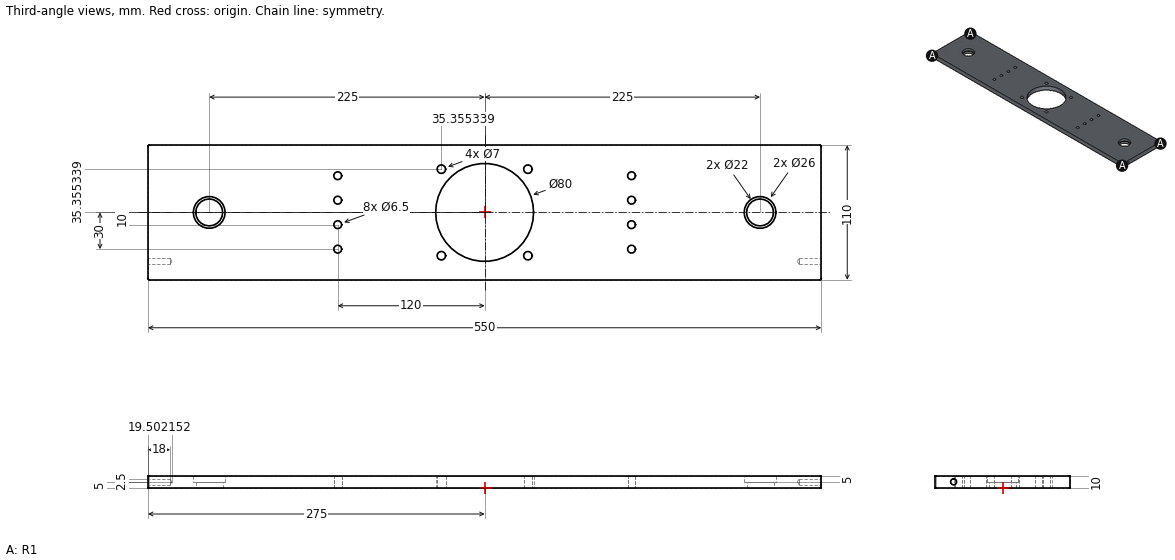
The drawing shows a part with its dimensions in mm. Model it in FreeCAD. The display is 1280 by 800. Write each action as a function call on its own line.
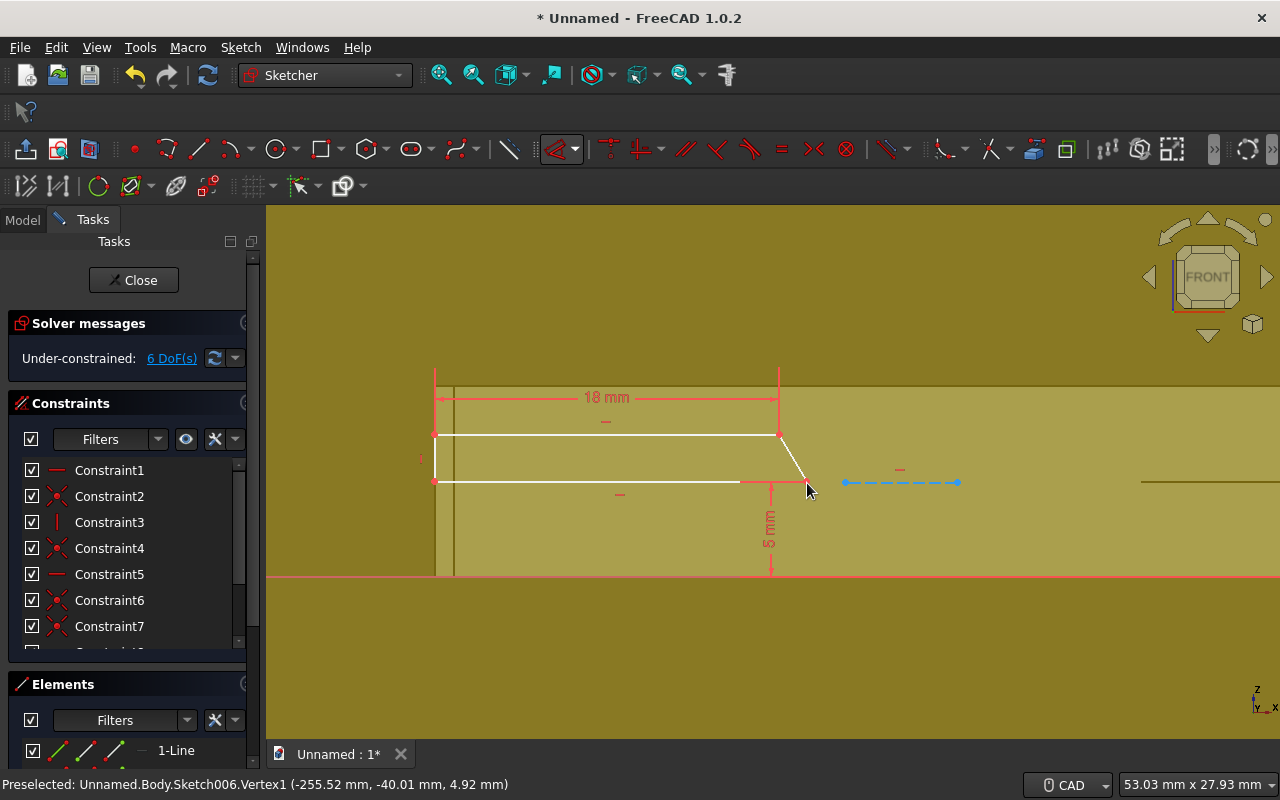
click(845, 483)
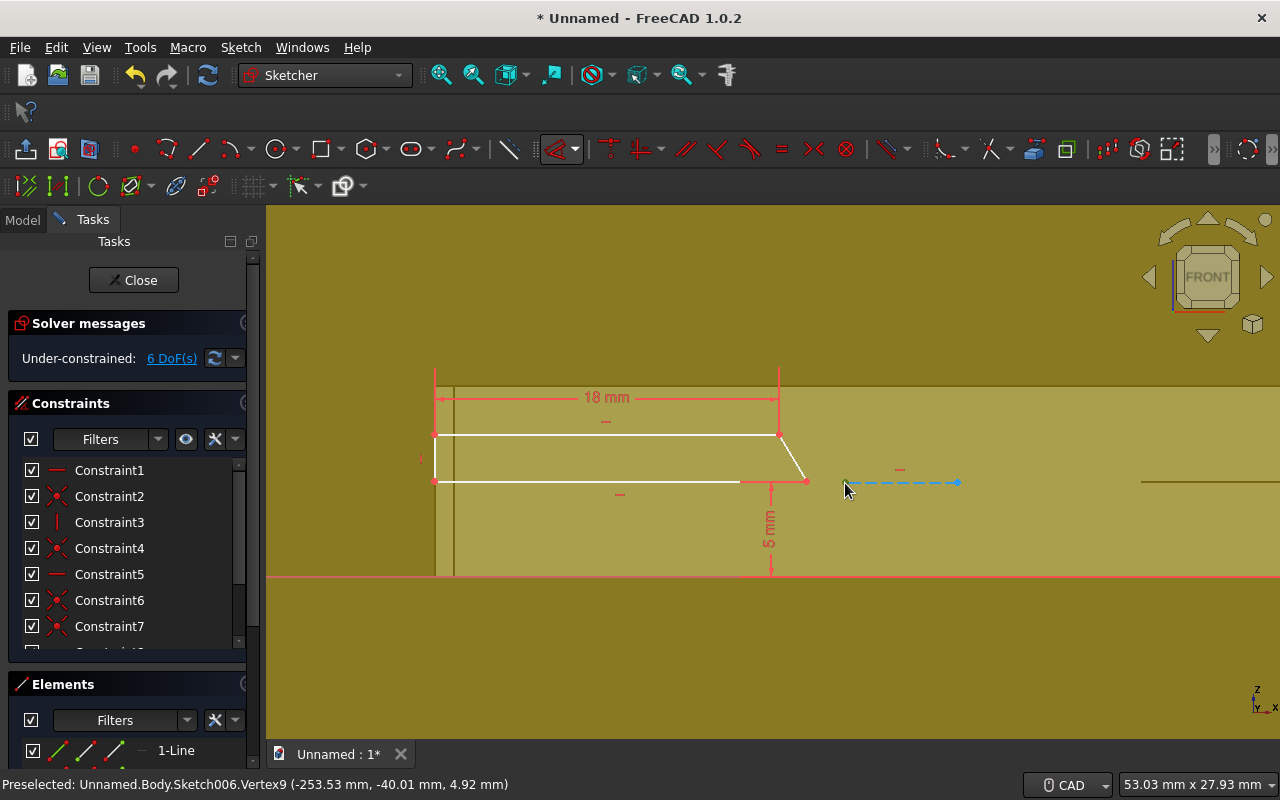
key(i)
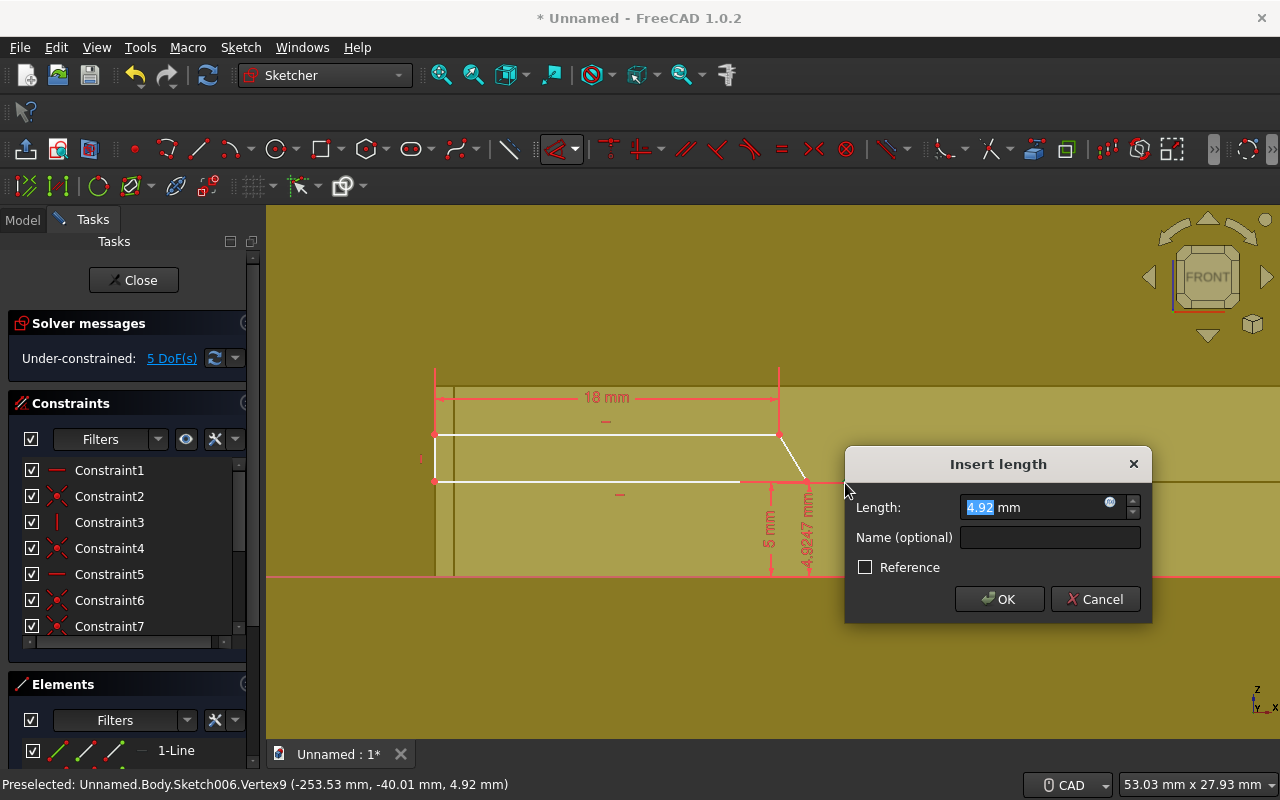
text(5)
key(Return)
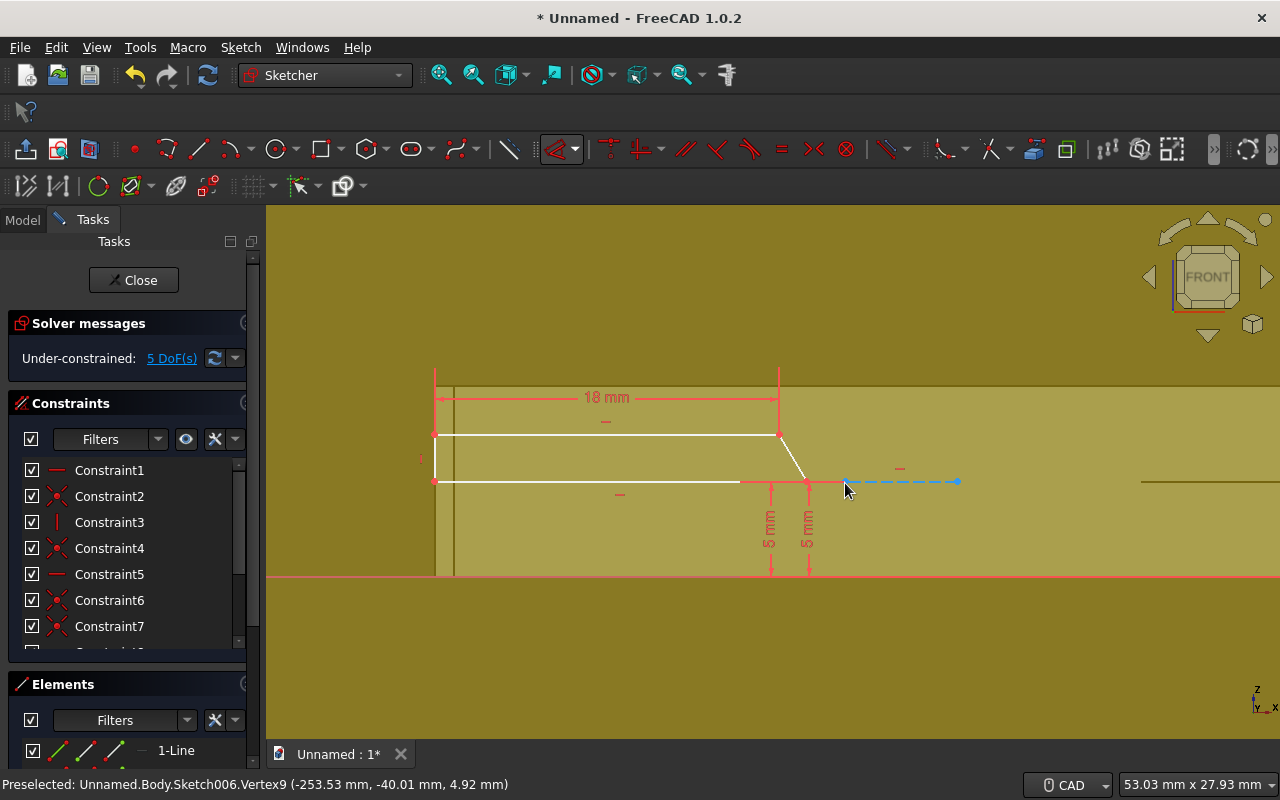
click(435, 468)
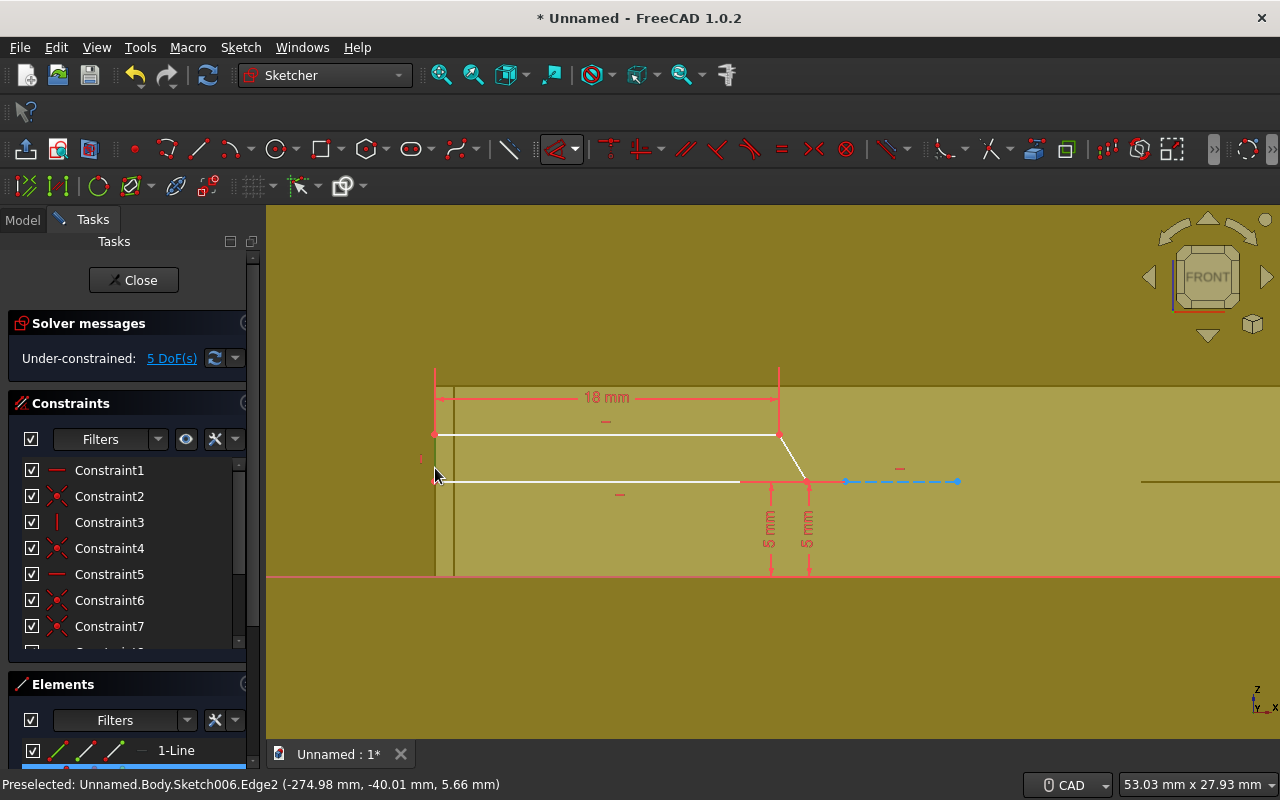
key(i)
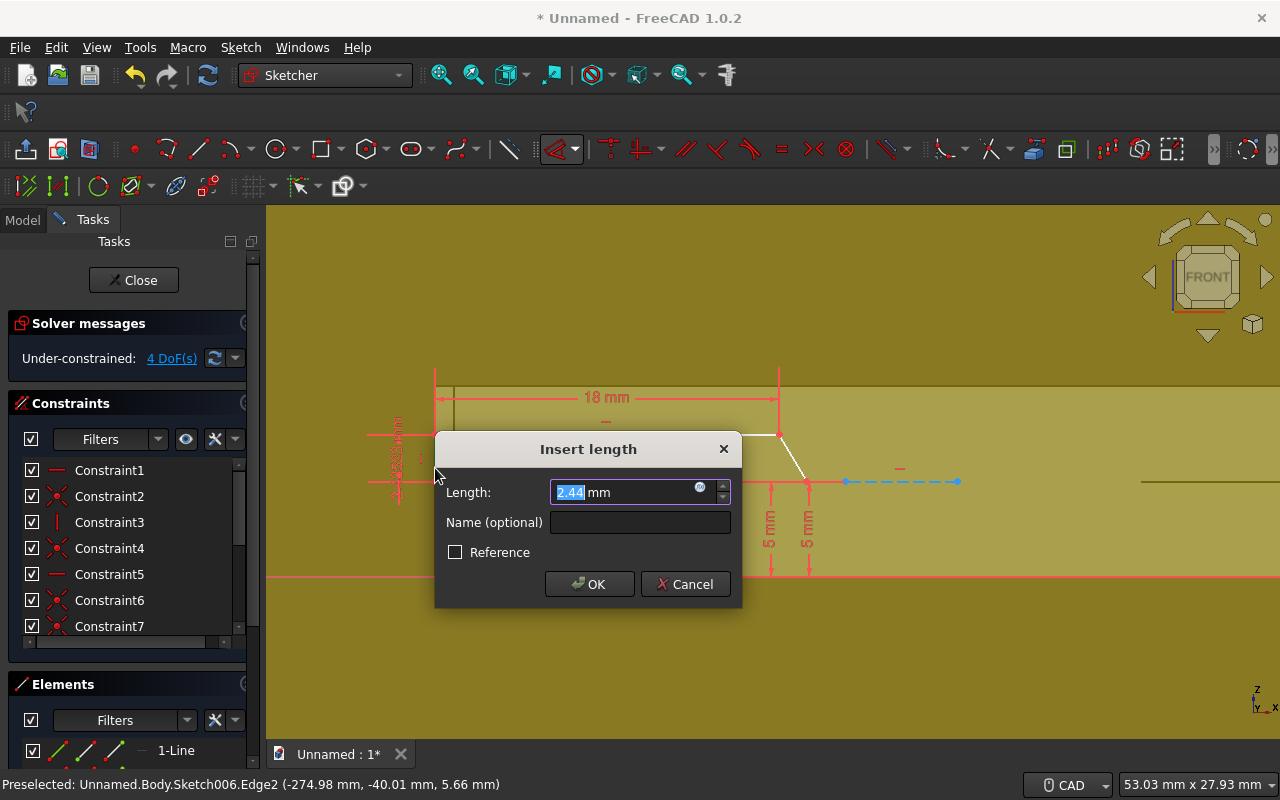
text(2.5)
key(Return)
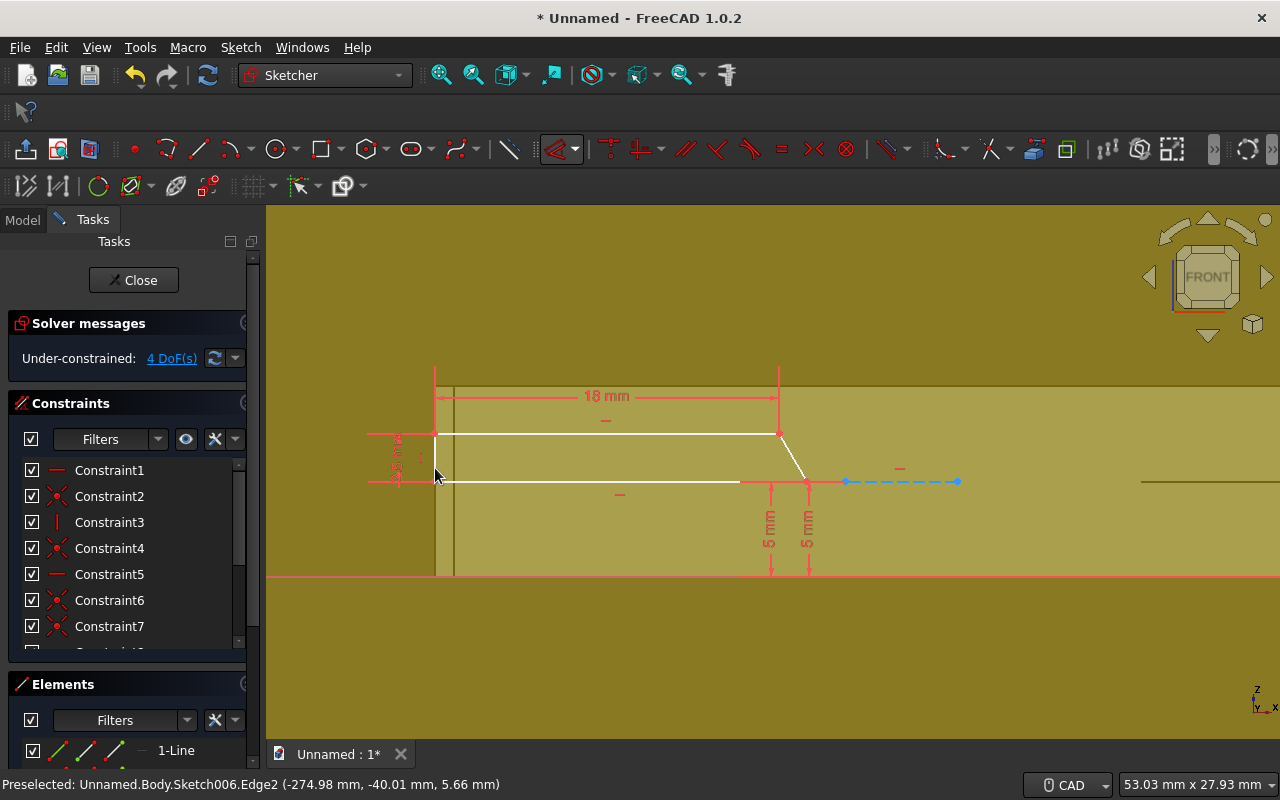
click(435, 482)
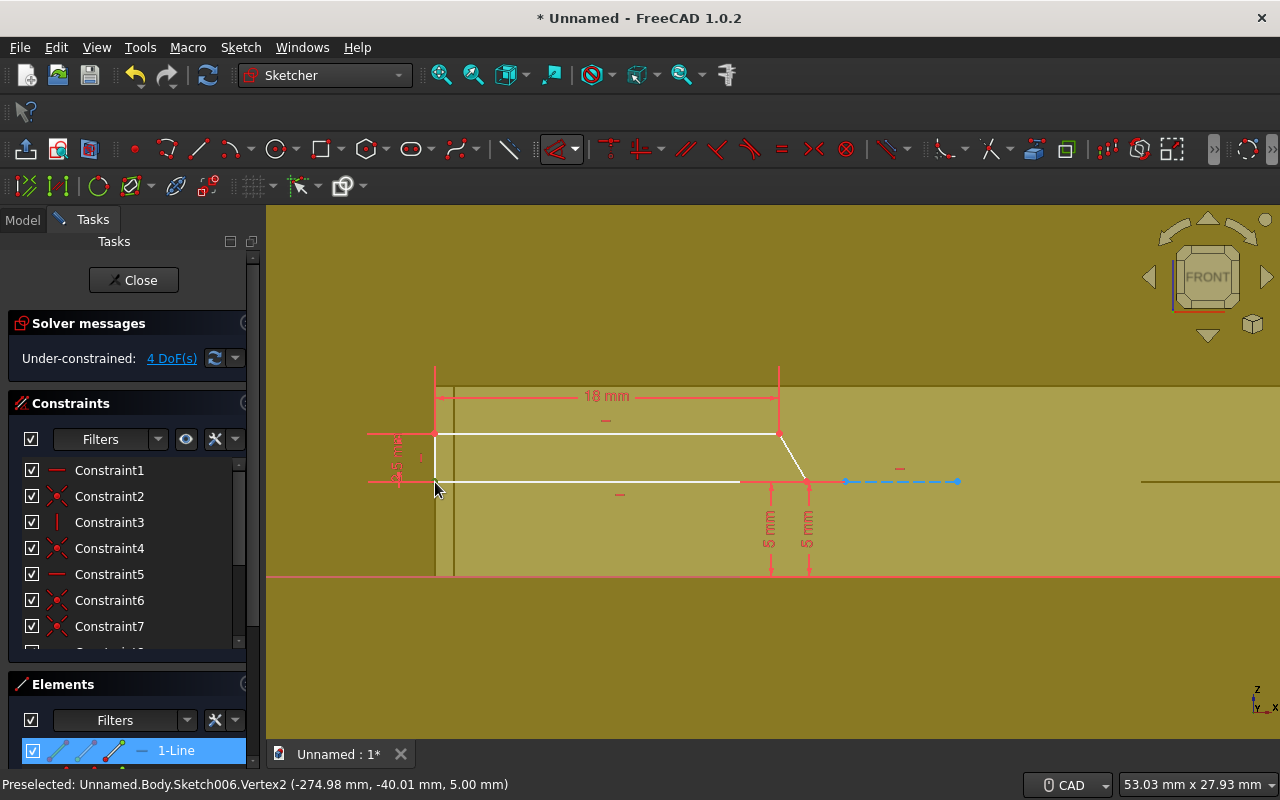
click(578, 150)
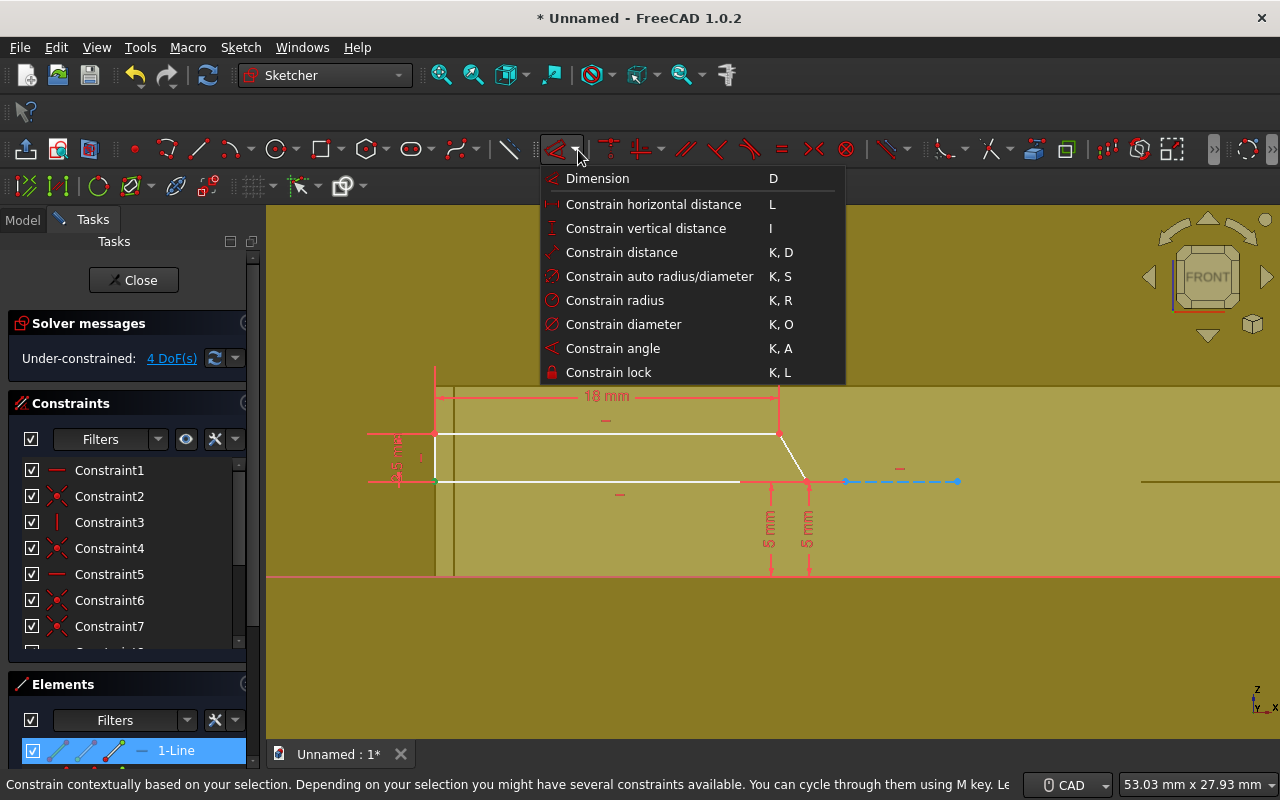
click(693, 204)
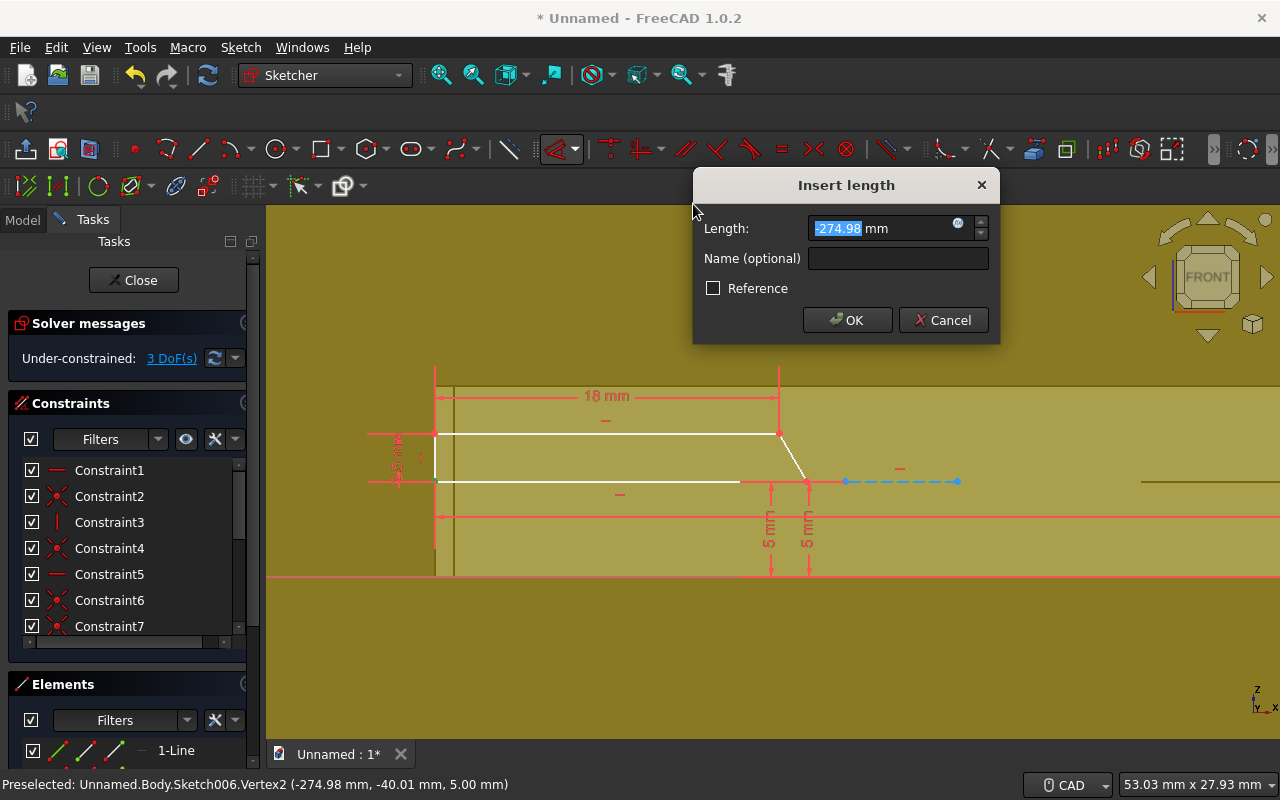
text(-275)
key(Return)